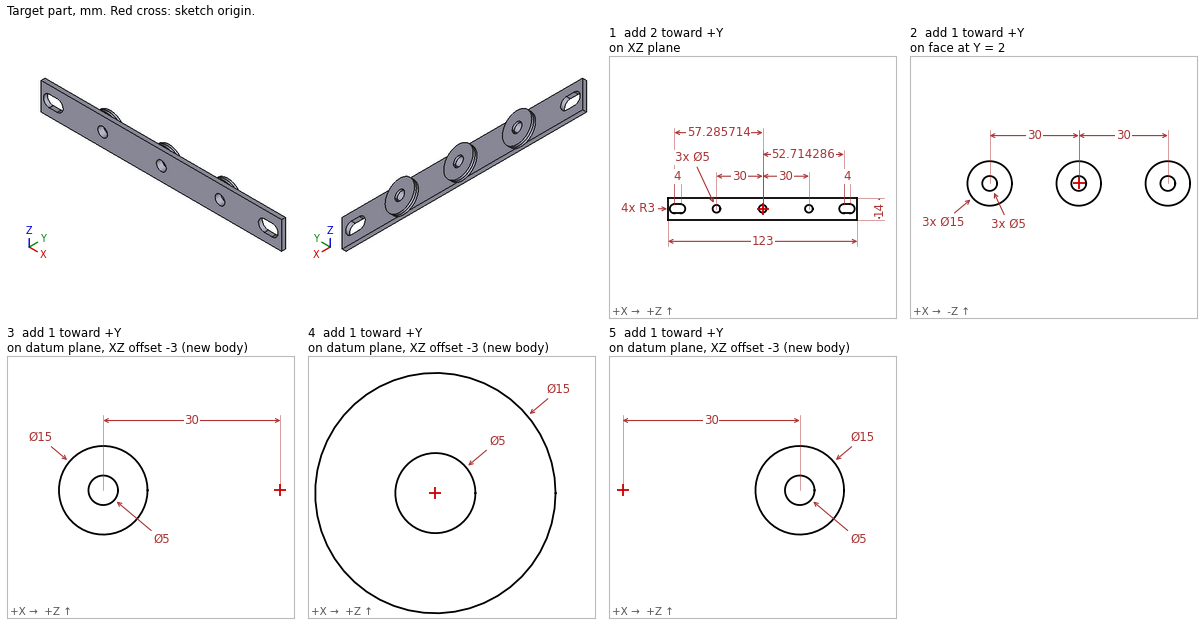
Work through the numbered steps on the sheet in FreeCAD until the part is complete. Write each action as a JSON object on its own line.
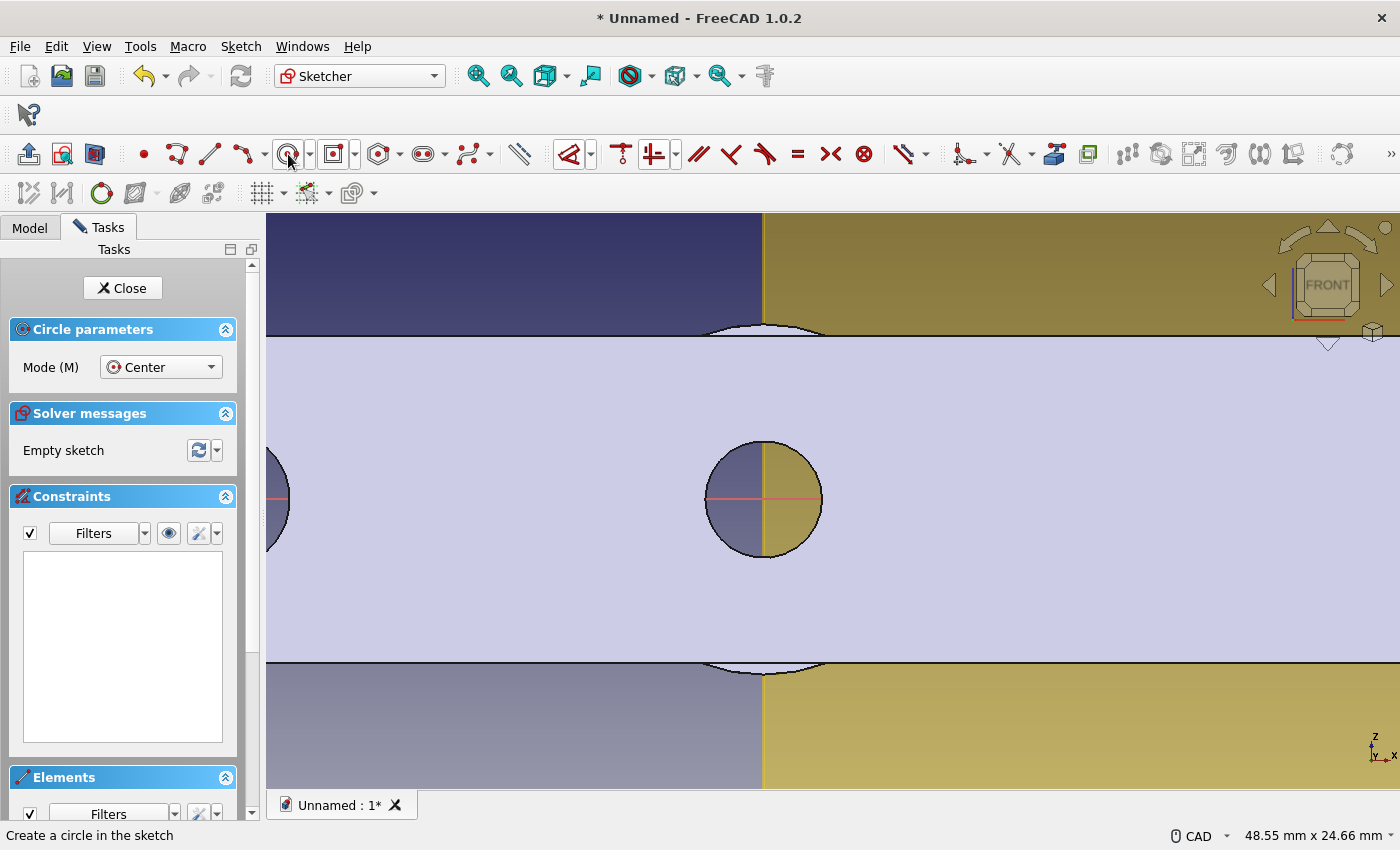
{"action": "left_click", "coordinate": [764, 499]}
{"action": "left_click", "coordinate": [888, 376]}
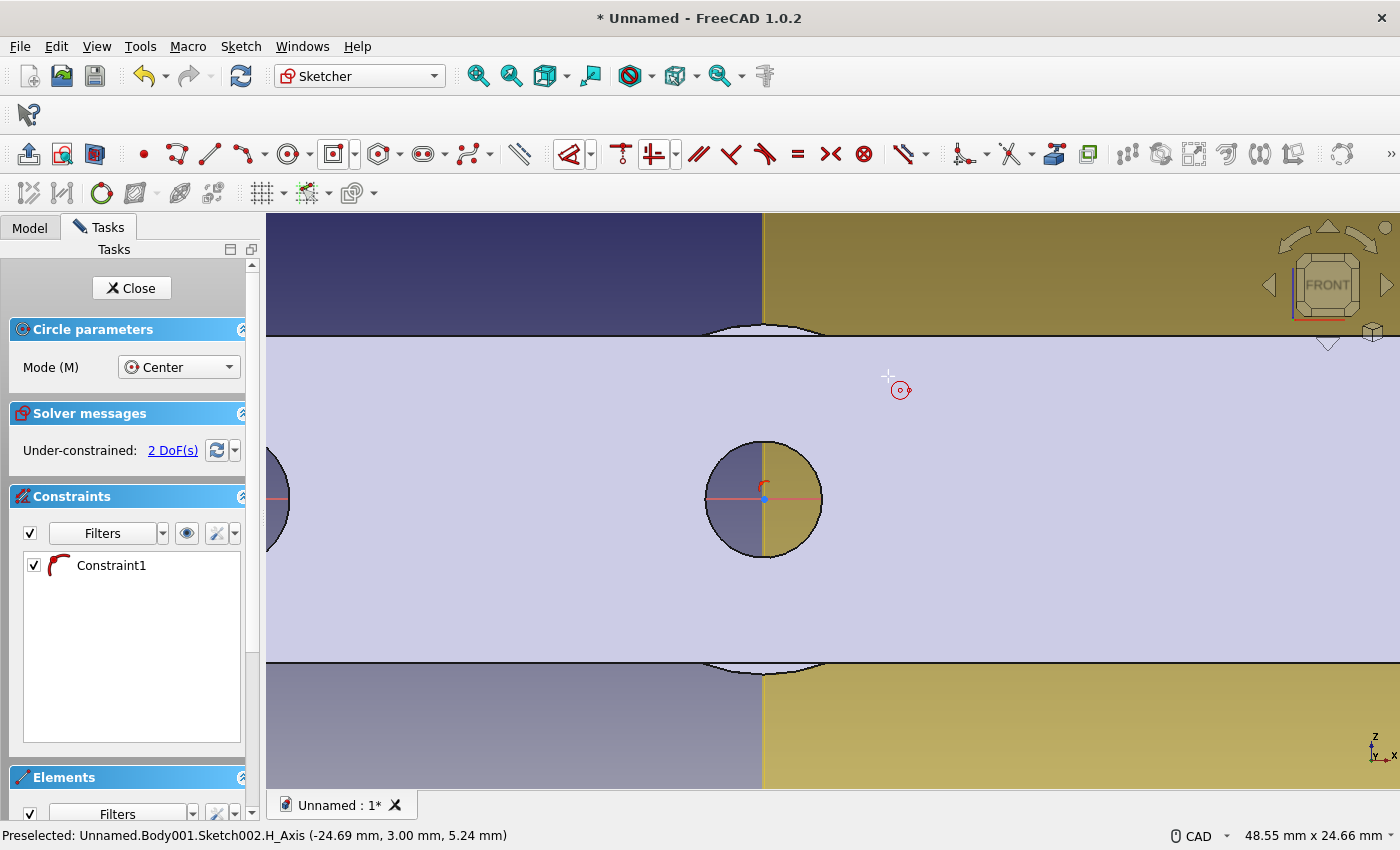
{"action": "left_click", "coordinate": [764, 499]}
{"action": "left_click", "coordinate": [805, 458]}
{"action": "key", "text": "Escape"}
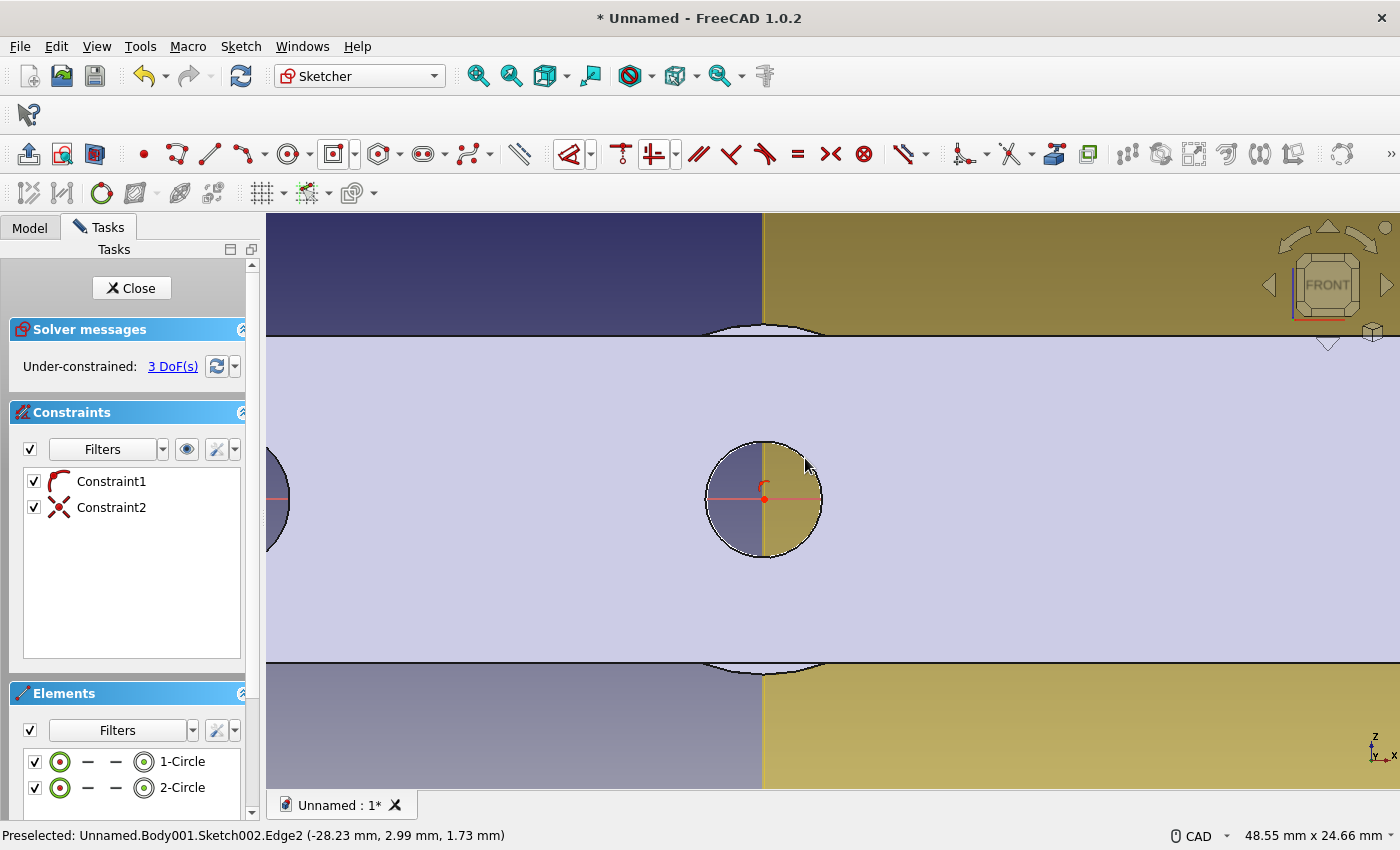
{"action": "left_click", "coordinate": [887, 376]}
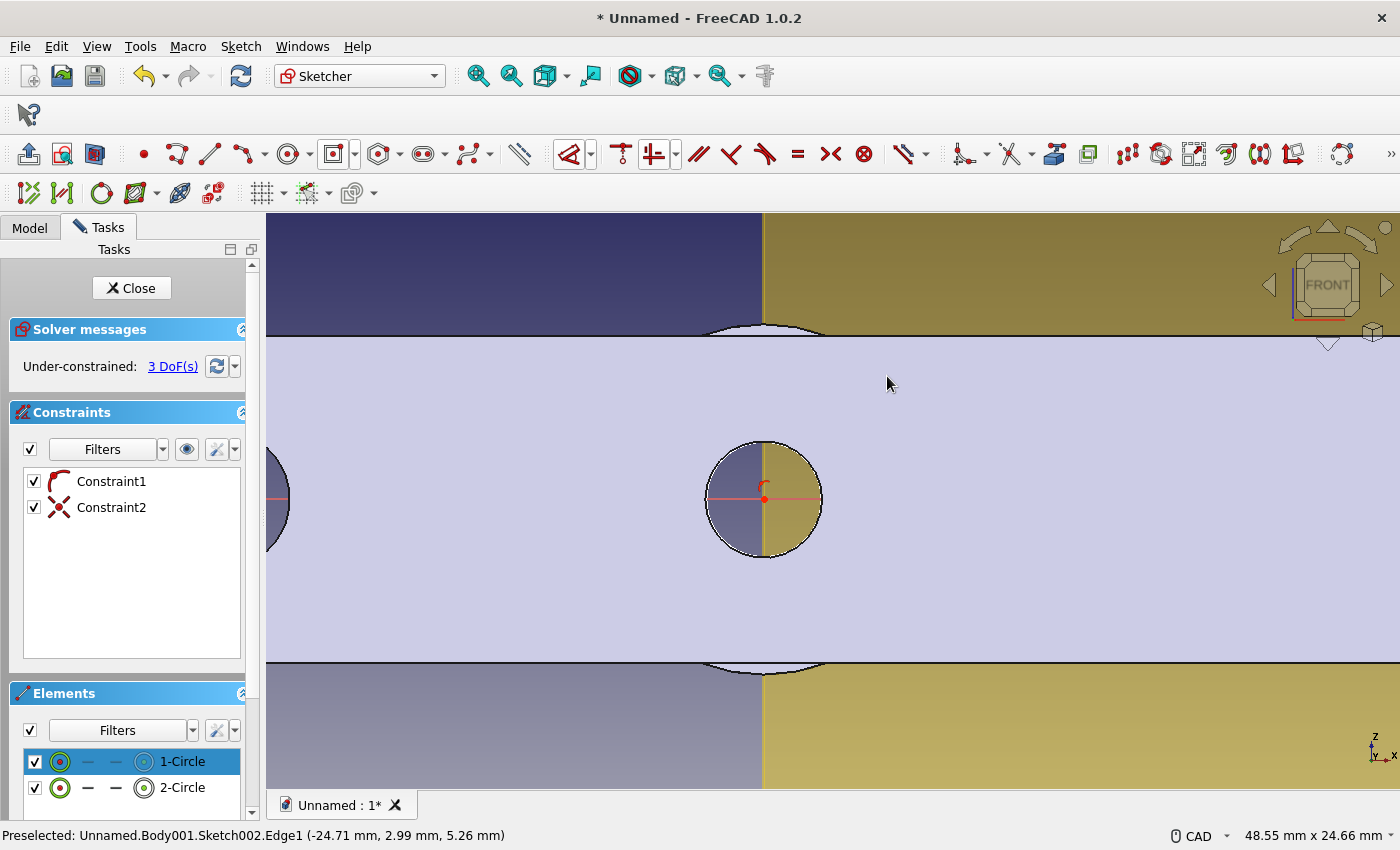
{"action": "left_click", "coordinate": [590, 154]}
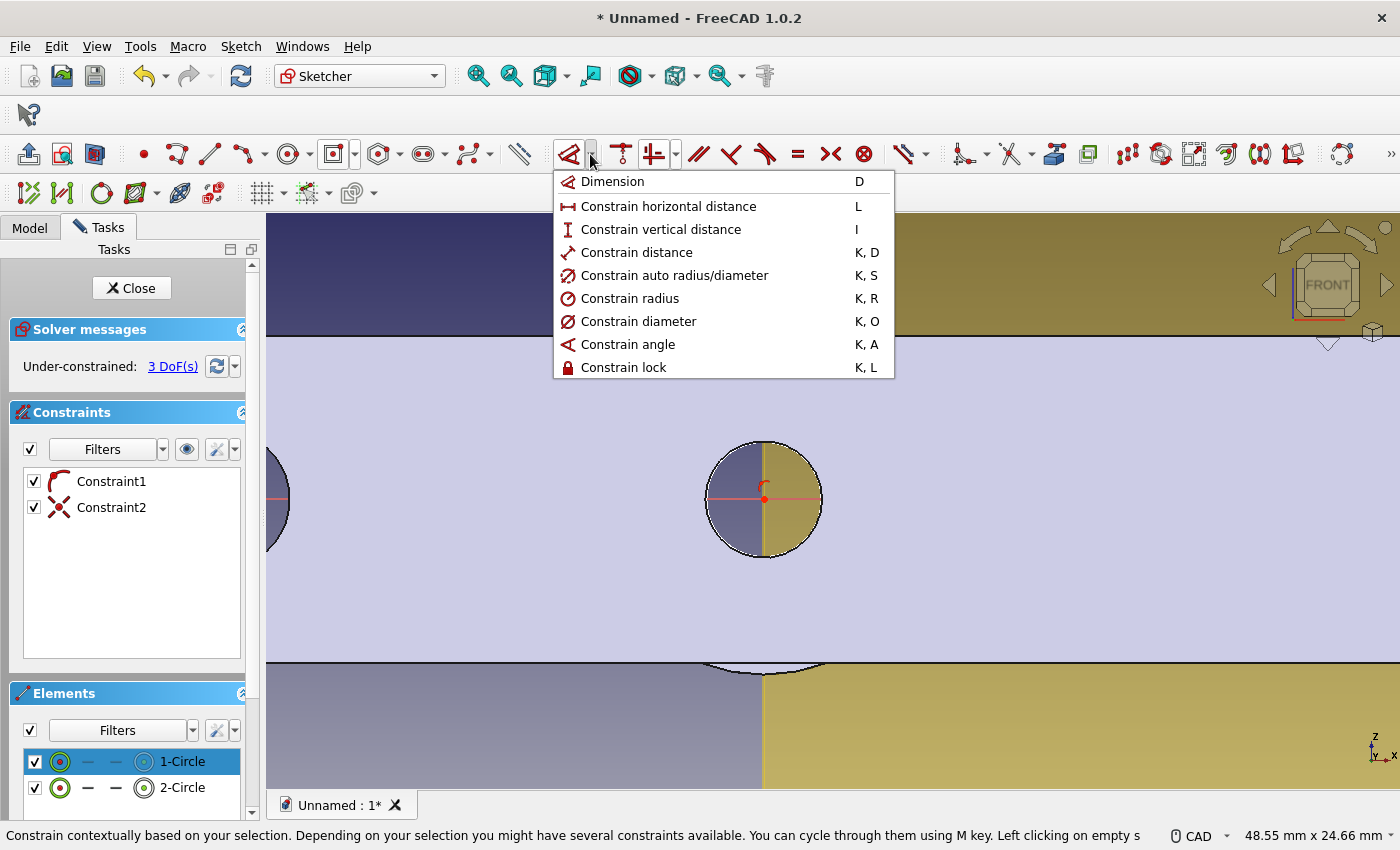
{"action": "left_click", "coordinate": [724, 322]}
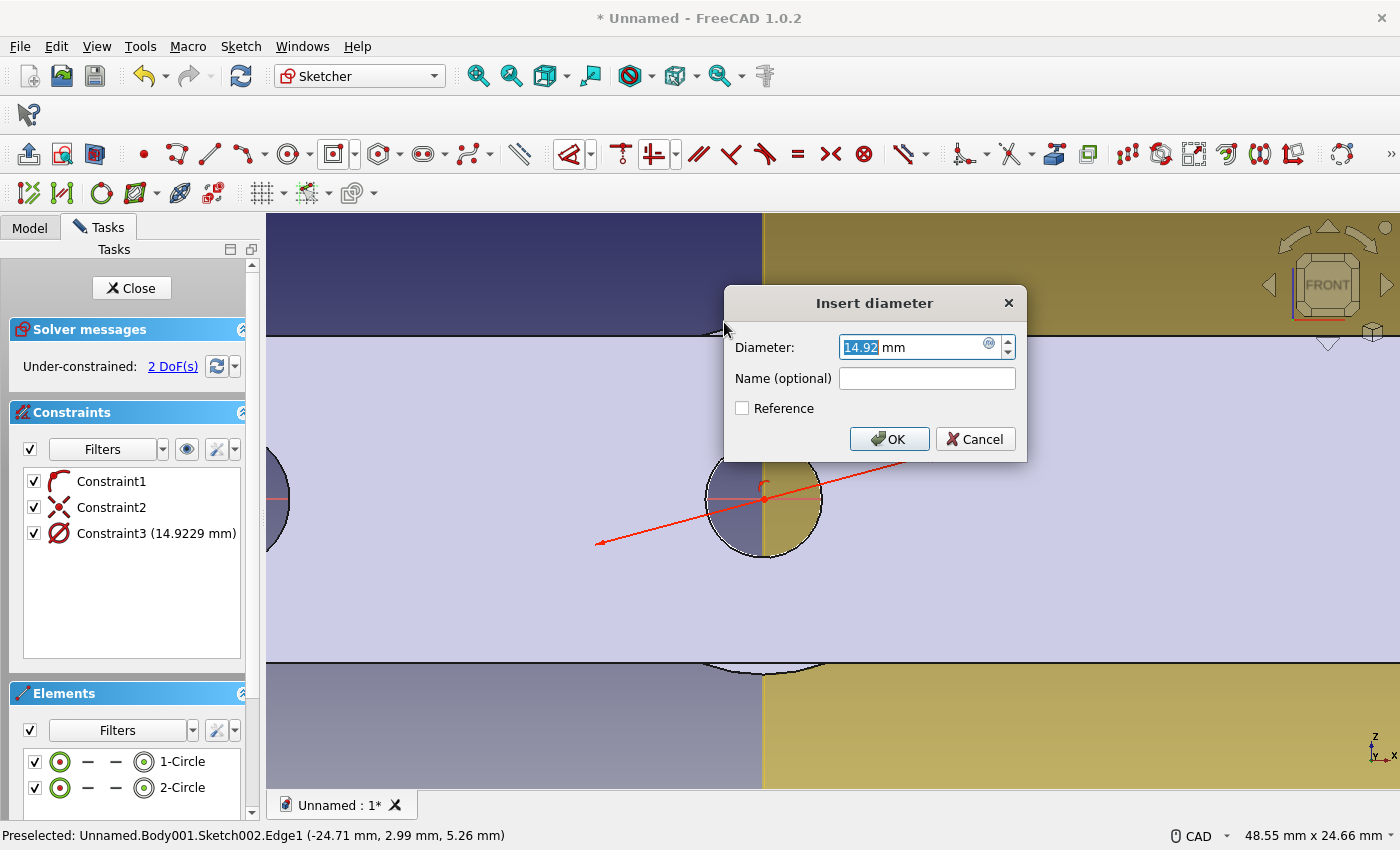
{"action": "type", "text": "15"}
{"action": "key", "text": "Return"}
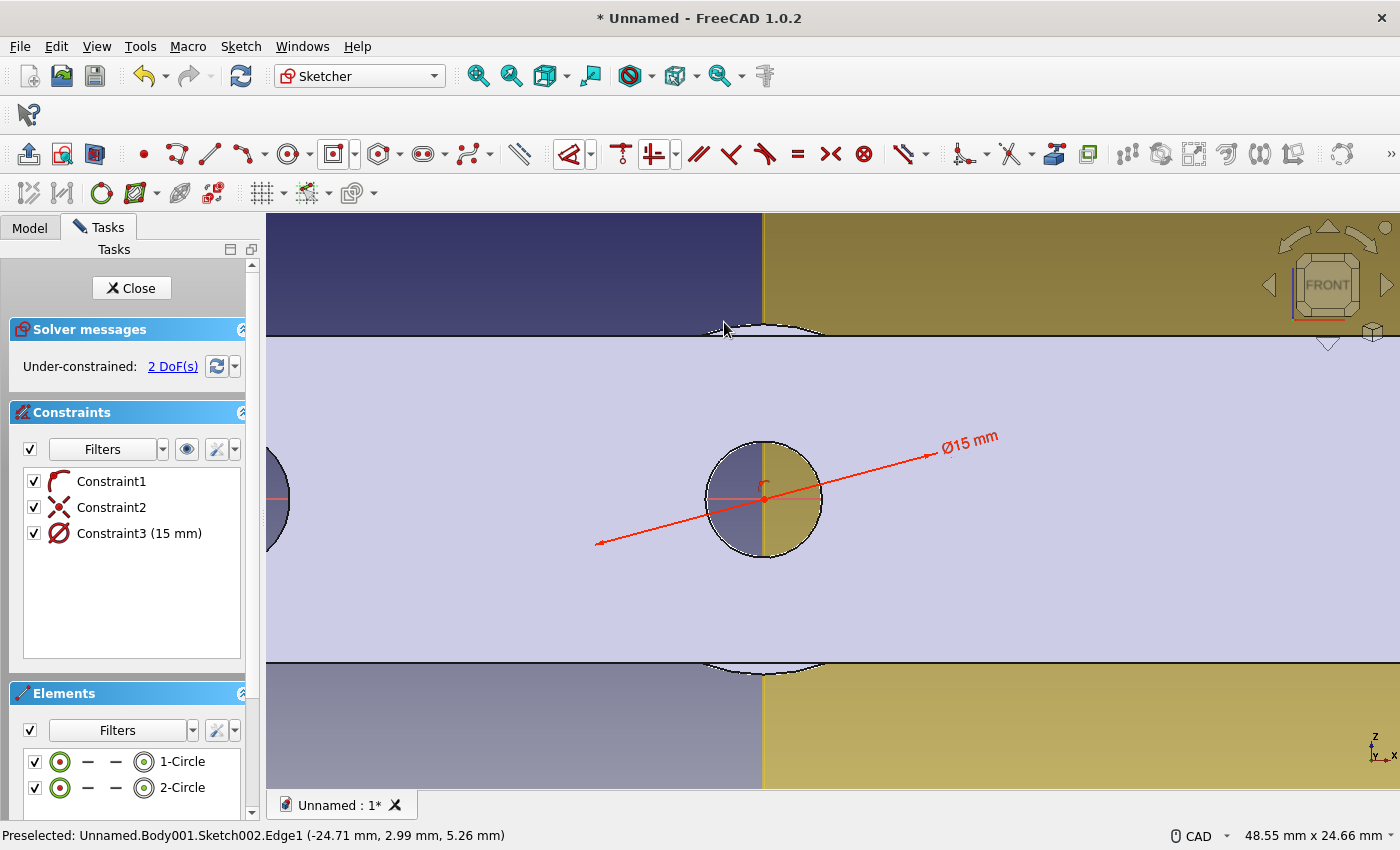
{"action": "left_click", "coordinate": [805, 459]}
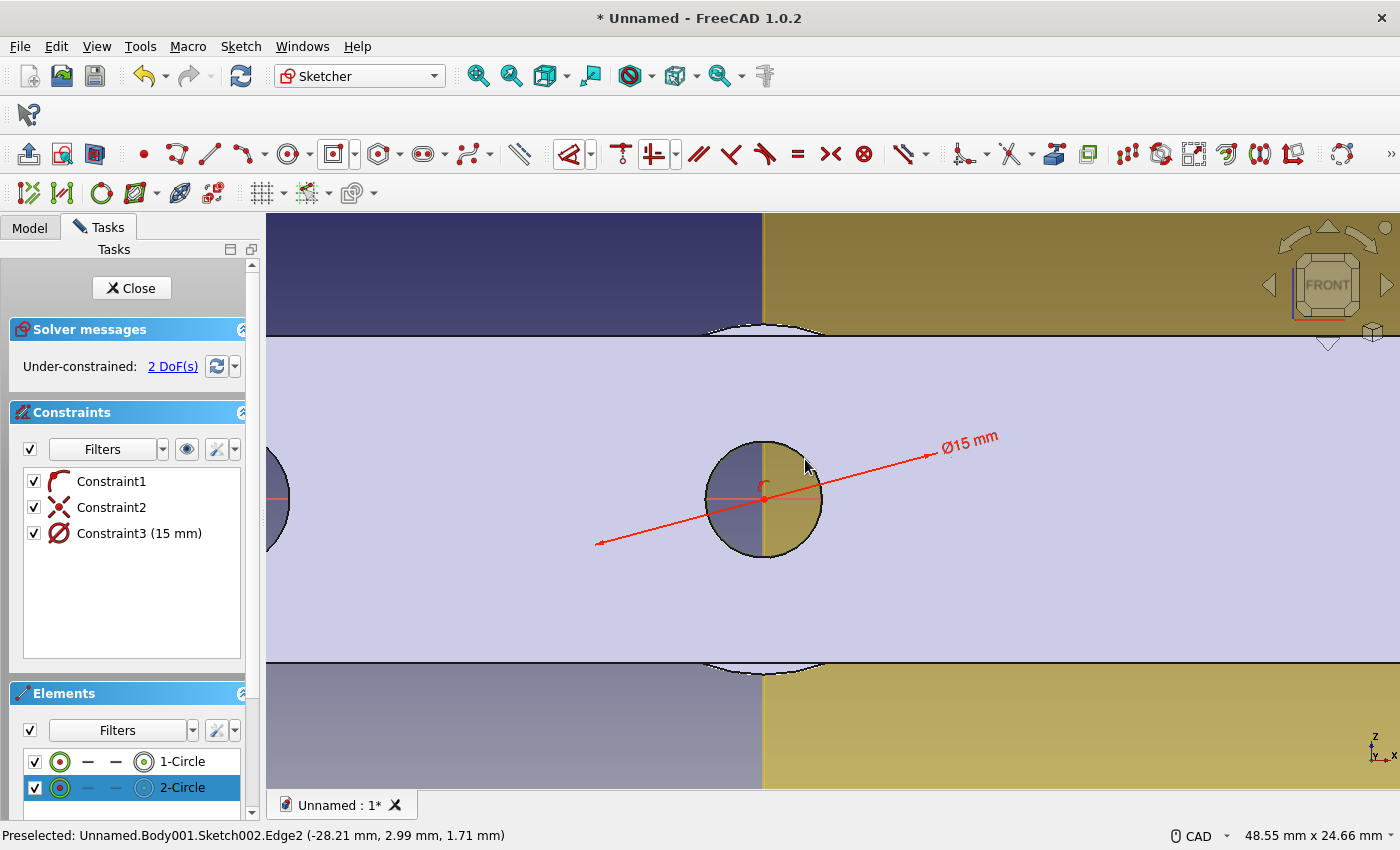
{"action": "key", "text": "k o"}